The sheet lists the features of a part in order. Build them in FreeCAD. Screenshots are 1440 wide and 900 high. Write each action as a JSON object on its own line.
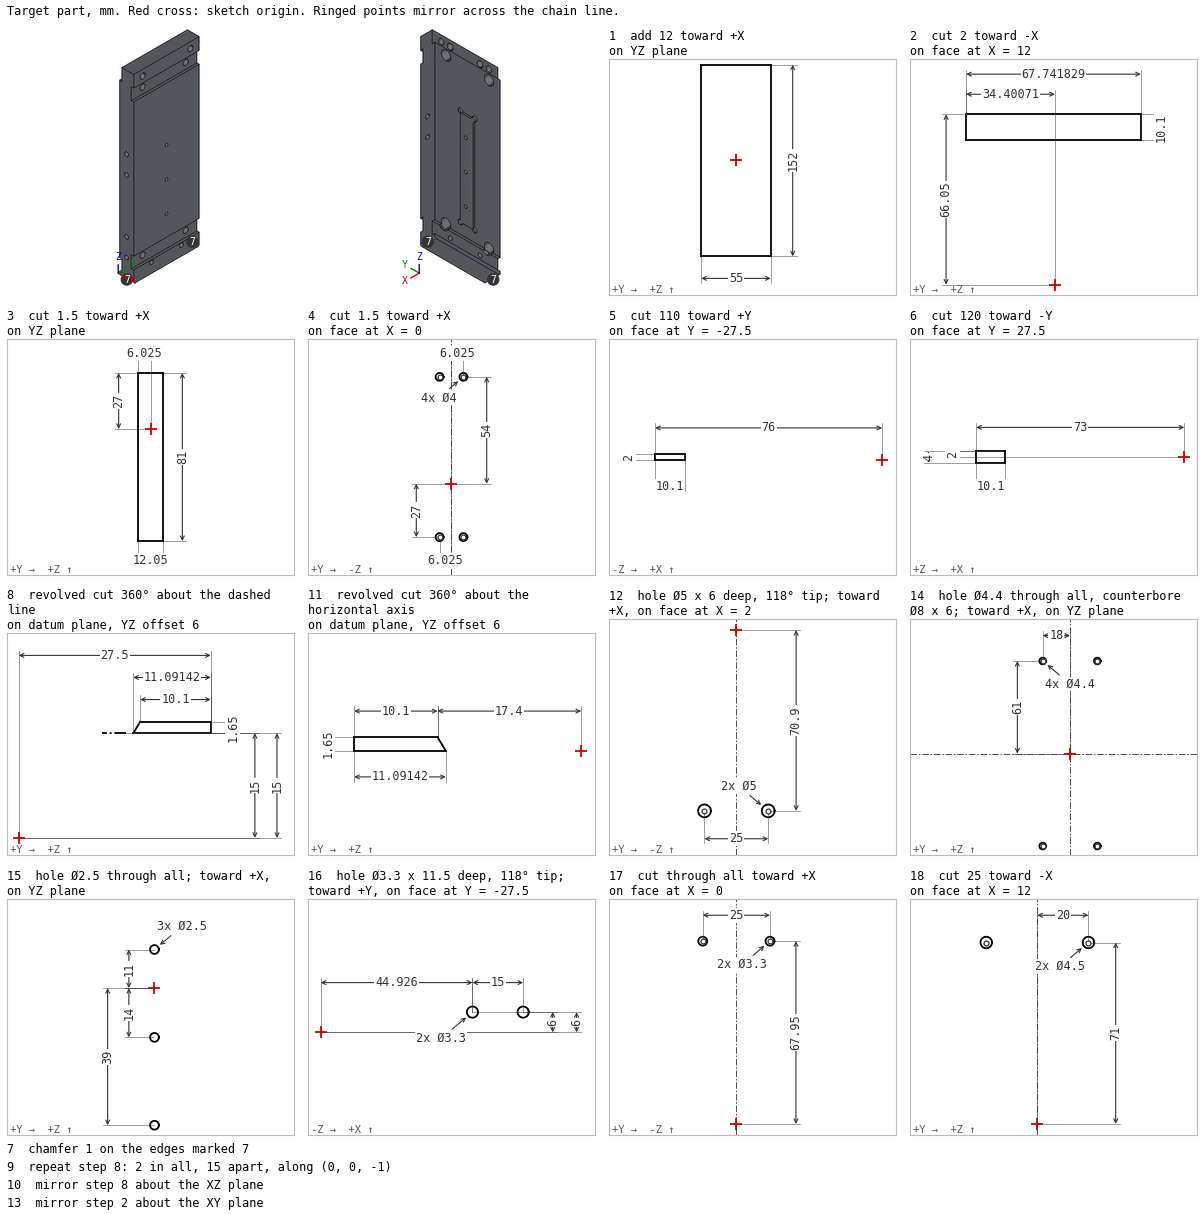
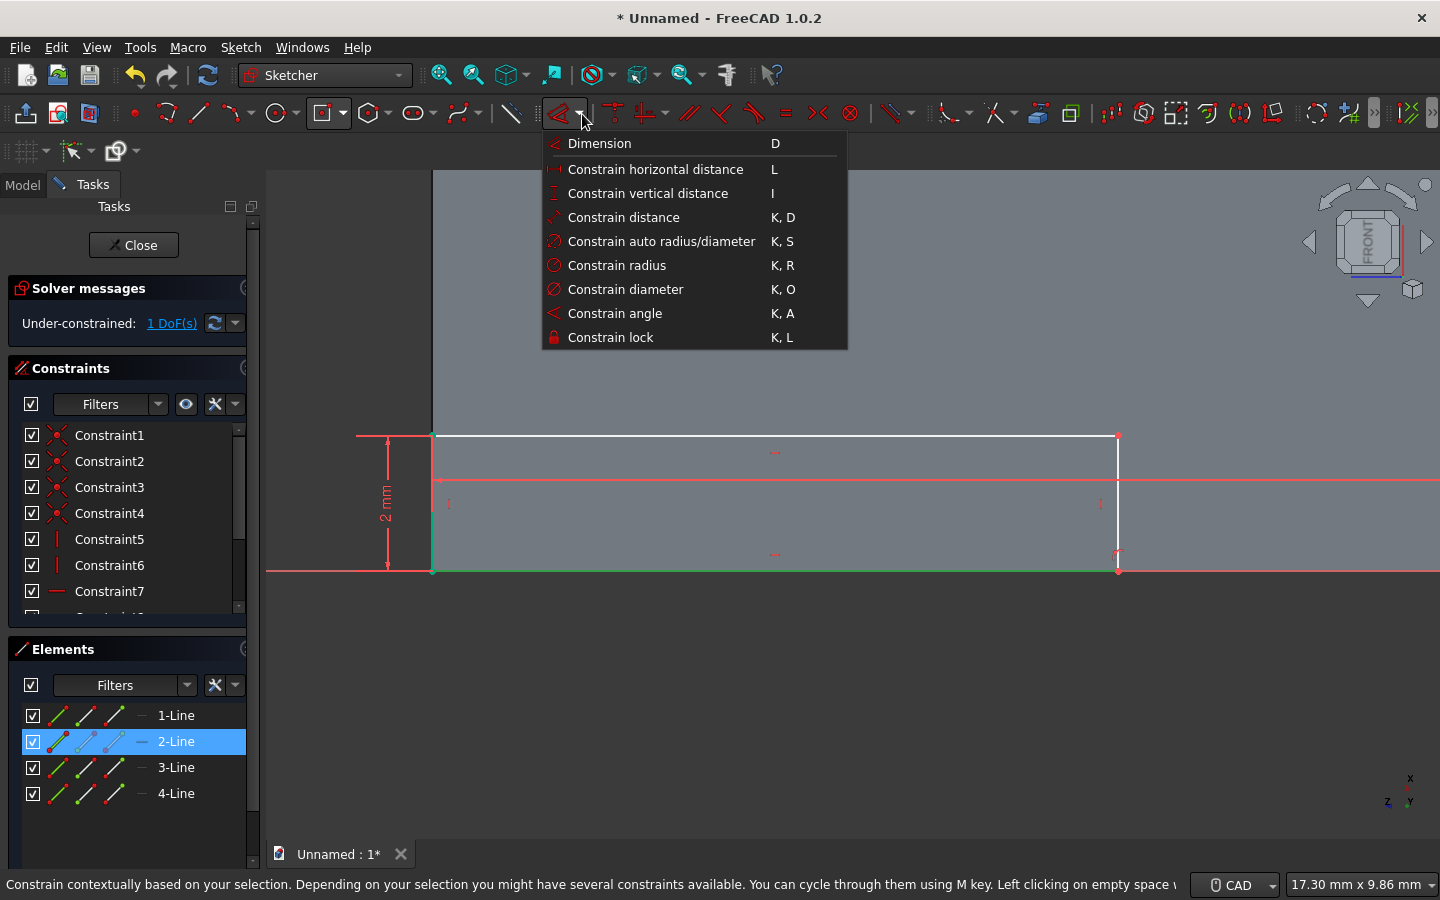
{"action": "left_click", "coordinate": [695, 169]}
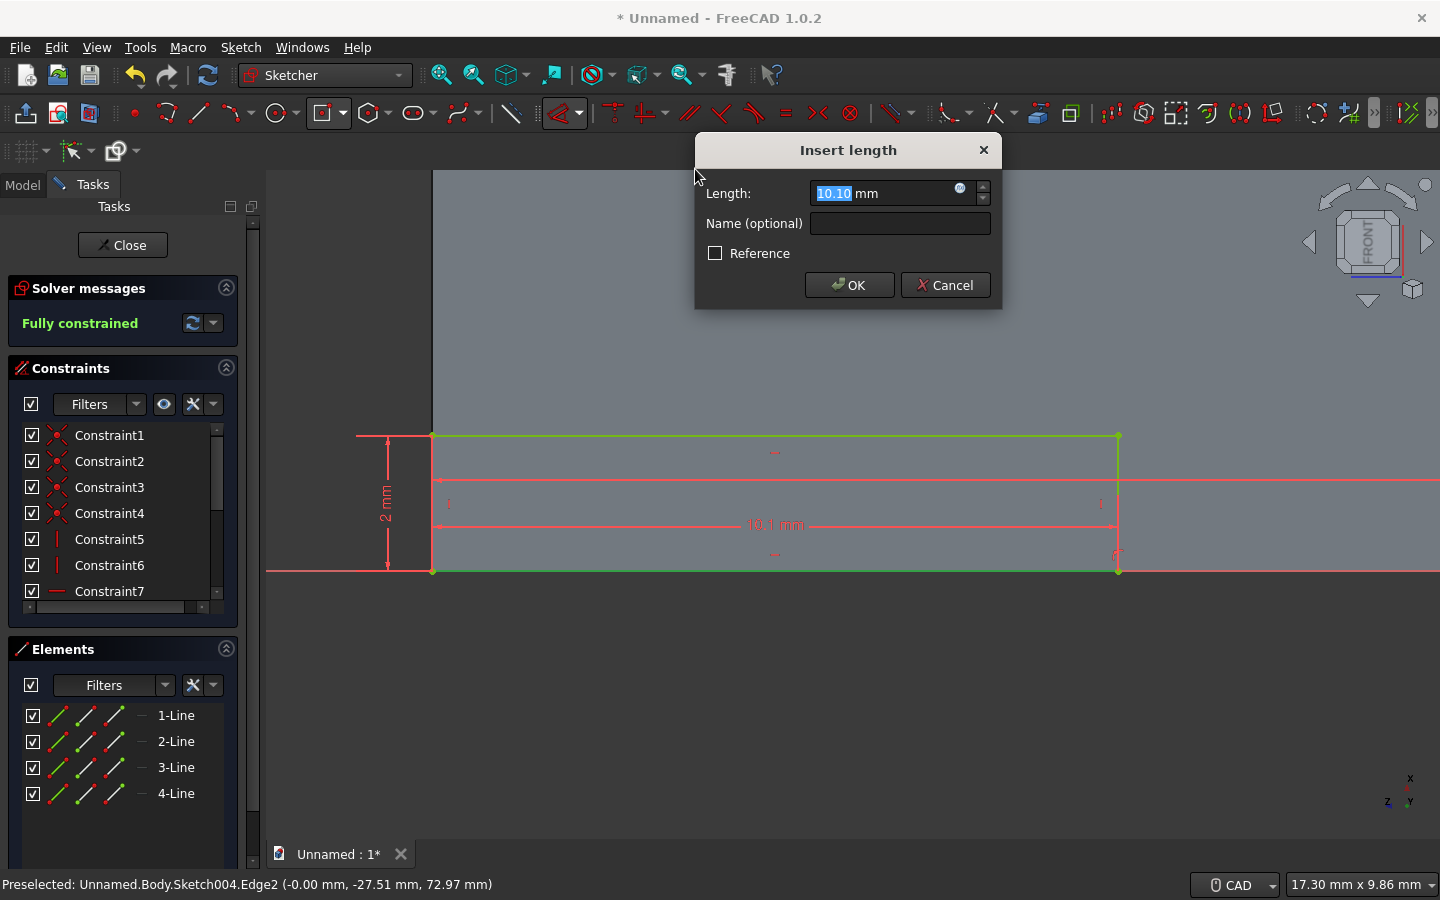
{"action": "type", "text": "10.1"}
{"action": "key", "text": "Return"}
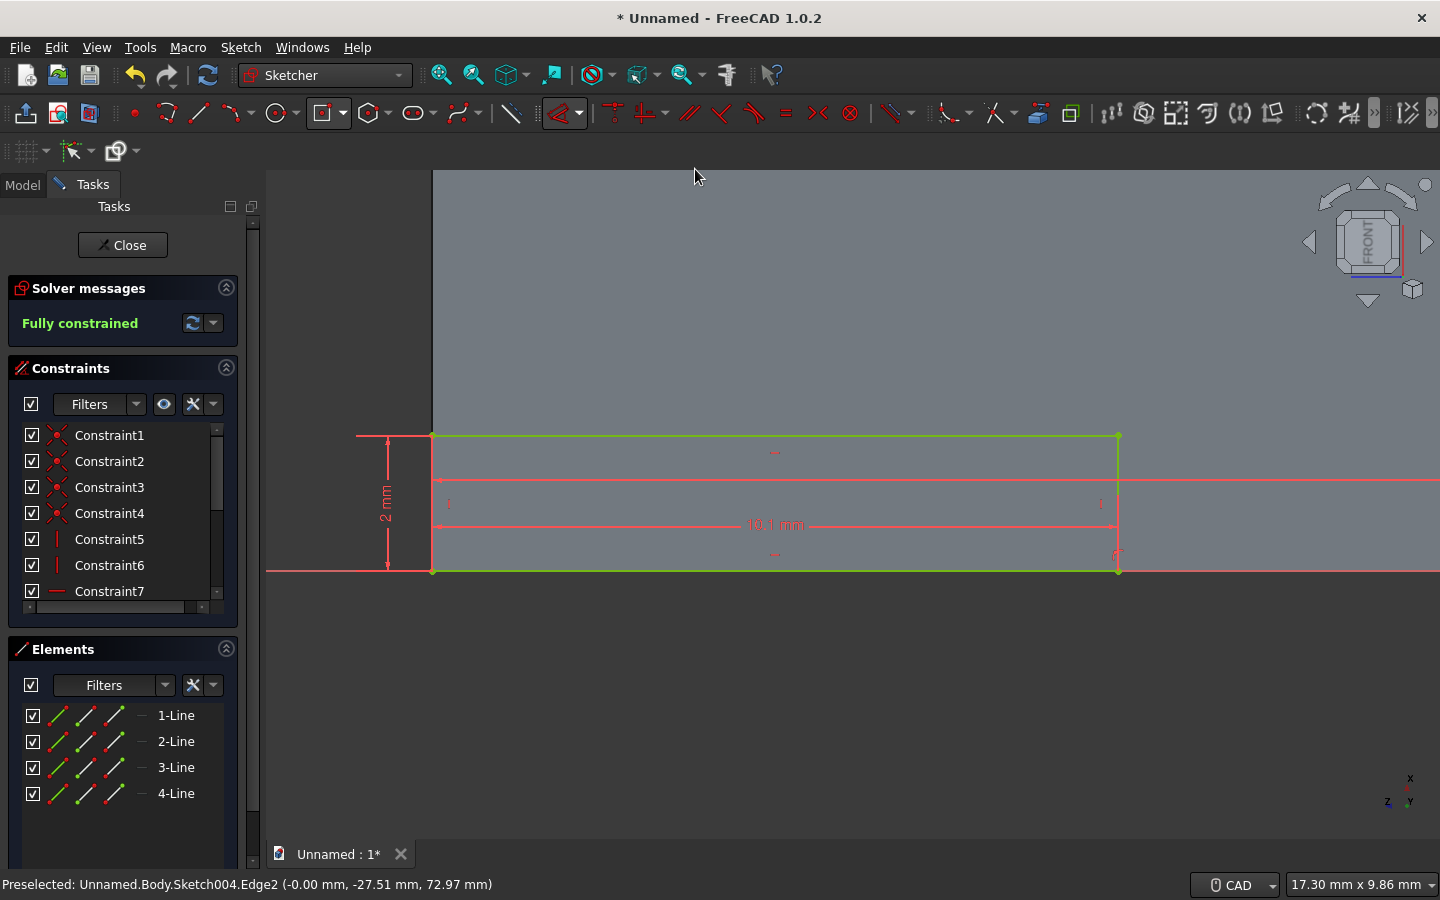
{"action": "left_click", "coordinate": [123, 245]}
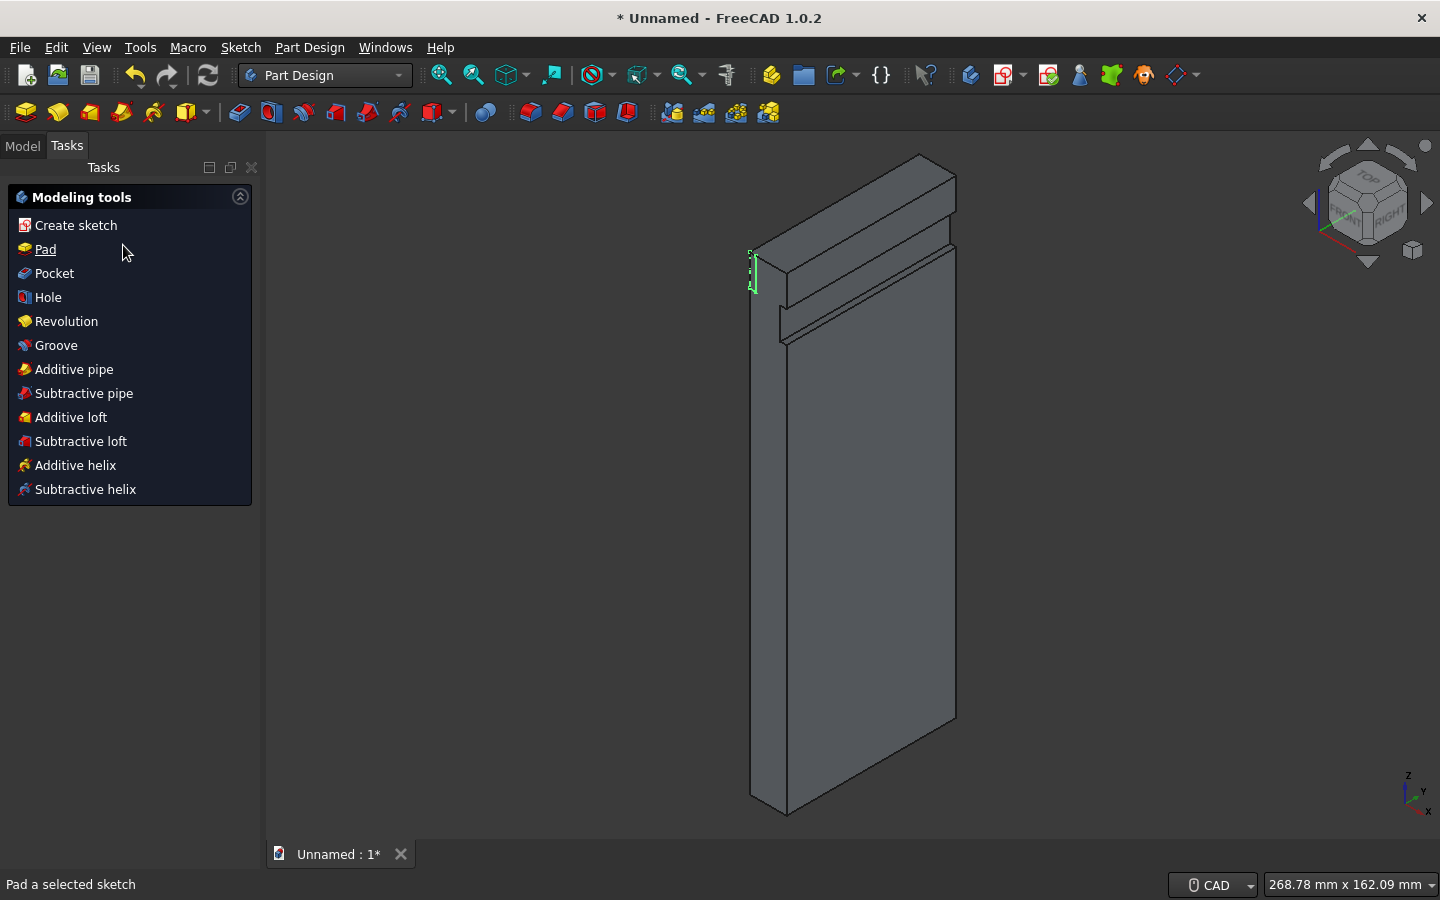
{"action": "left_click", "coordinate": [240, 112]}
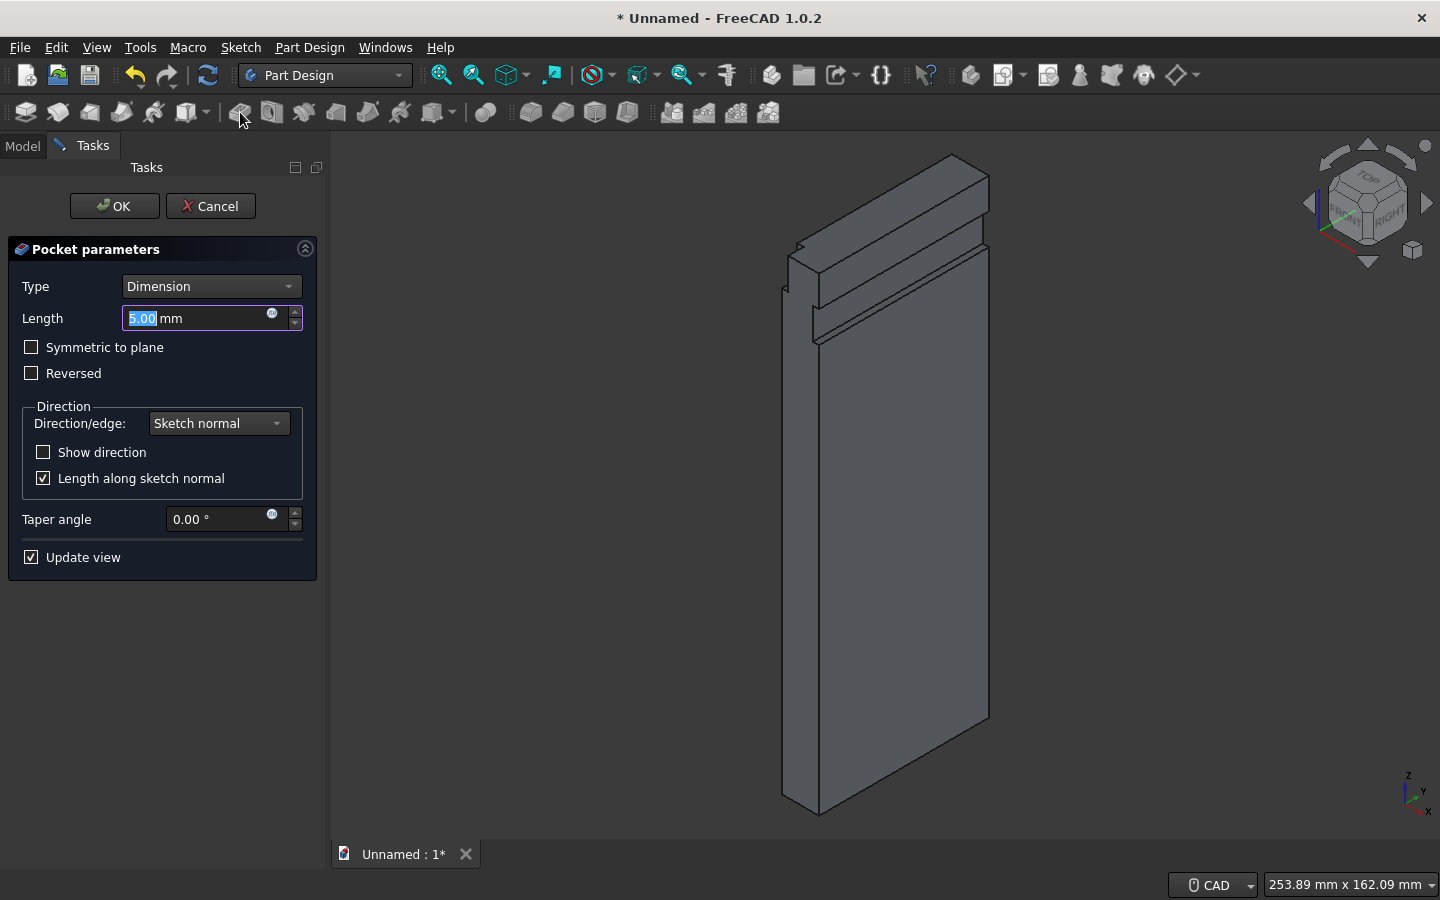
{"action": "type", "text": "110"}
{"action": "key", "text": "Tab"}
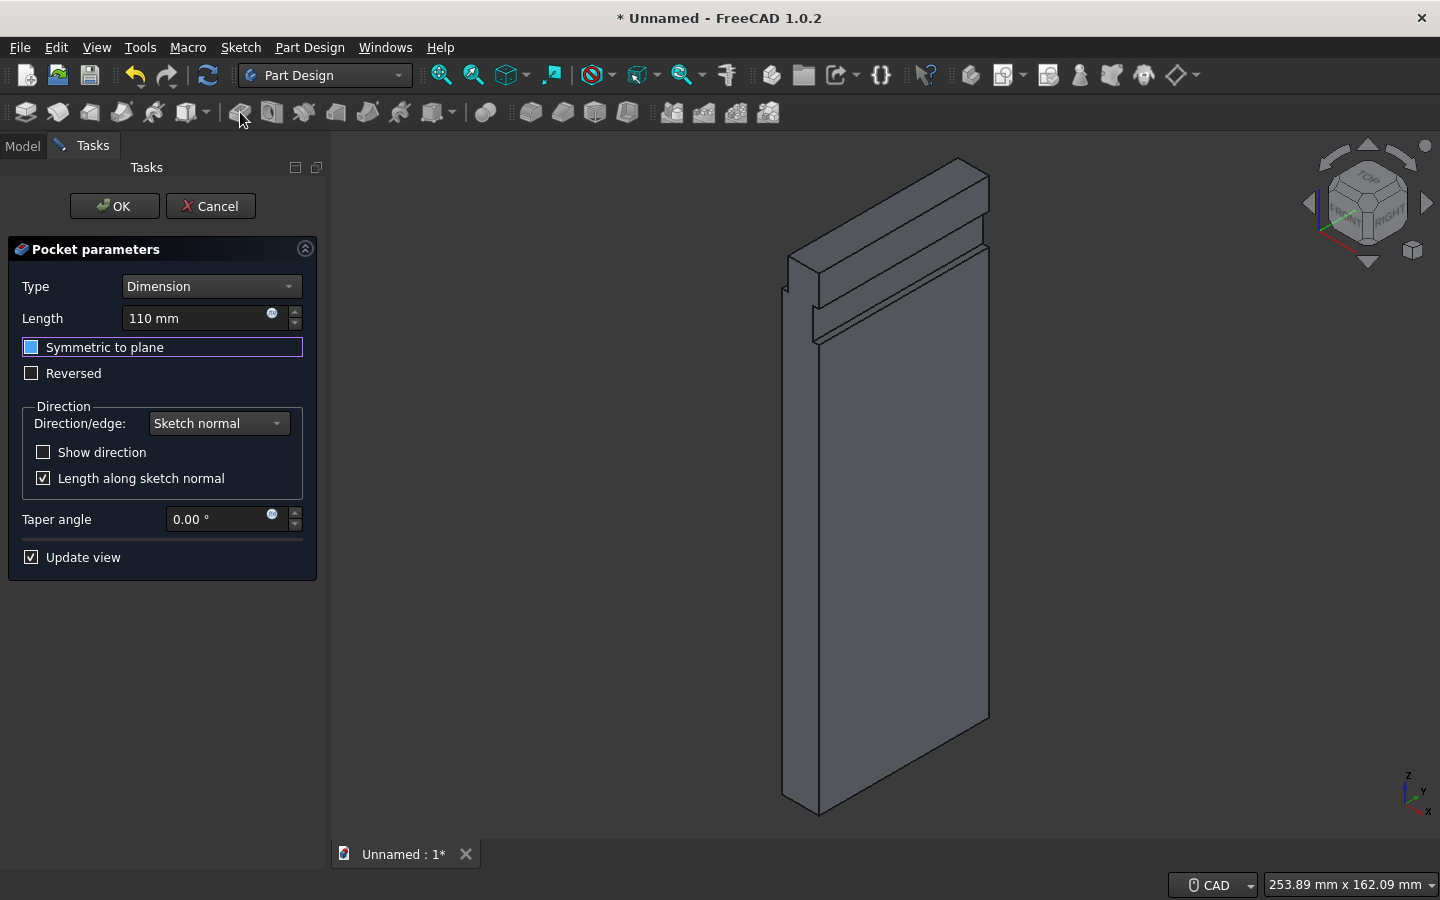
{"action": "left_click", "coordinate": [115, 206]}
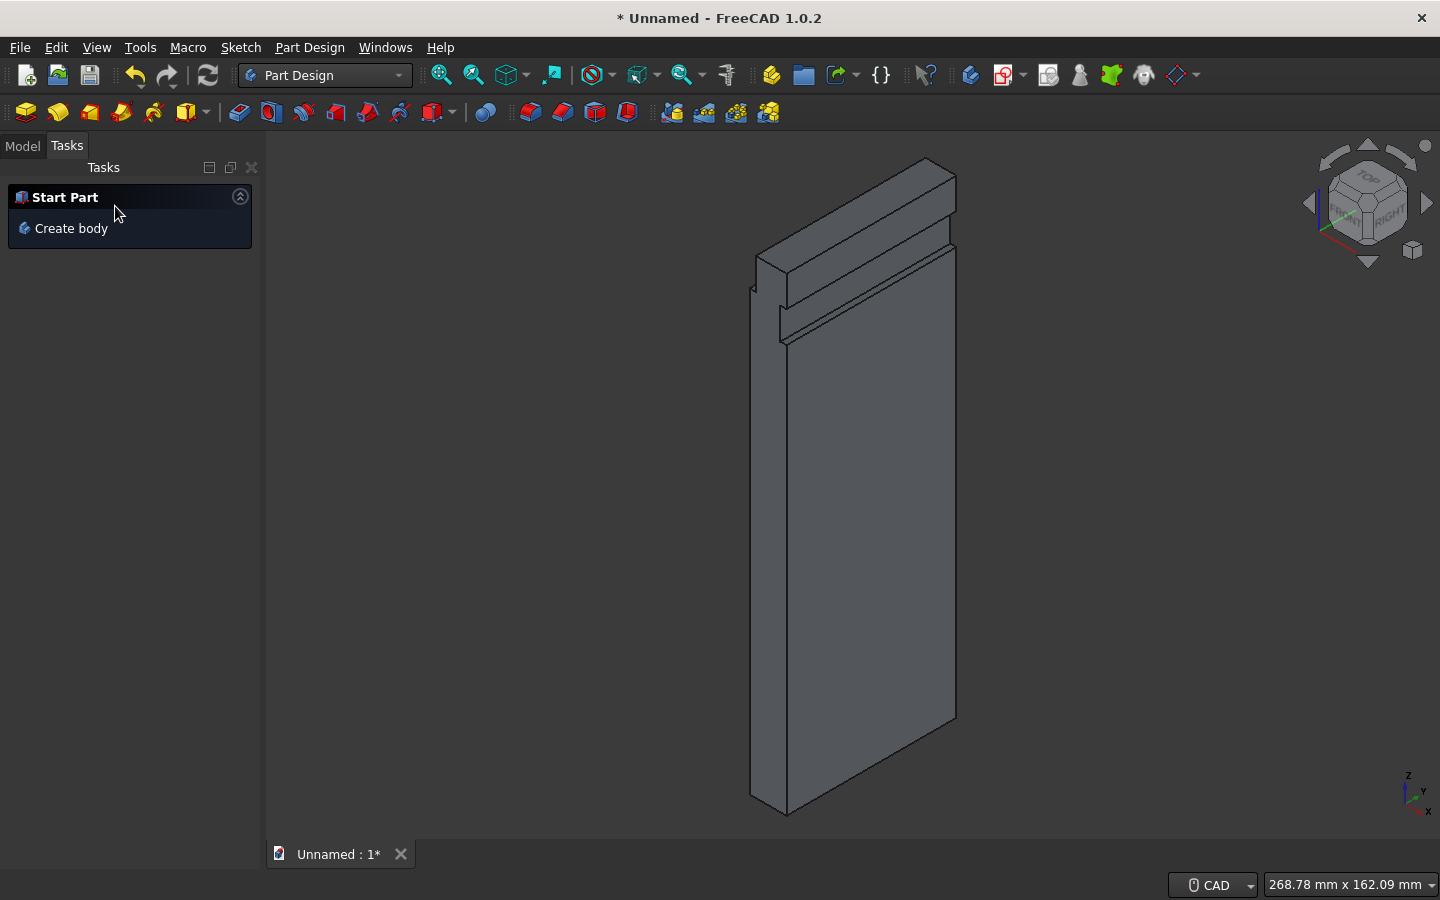
{"action": "key", "text": "4"}